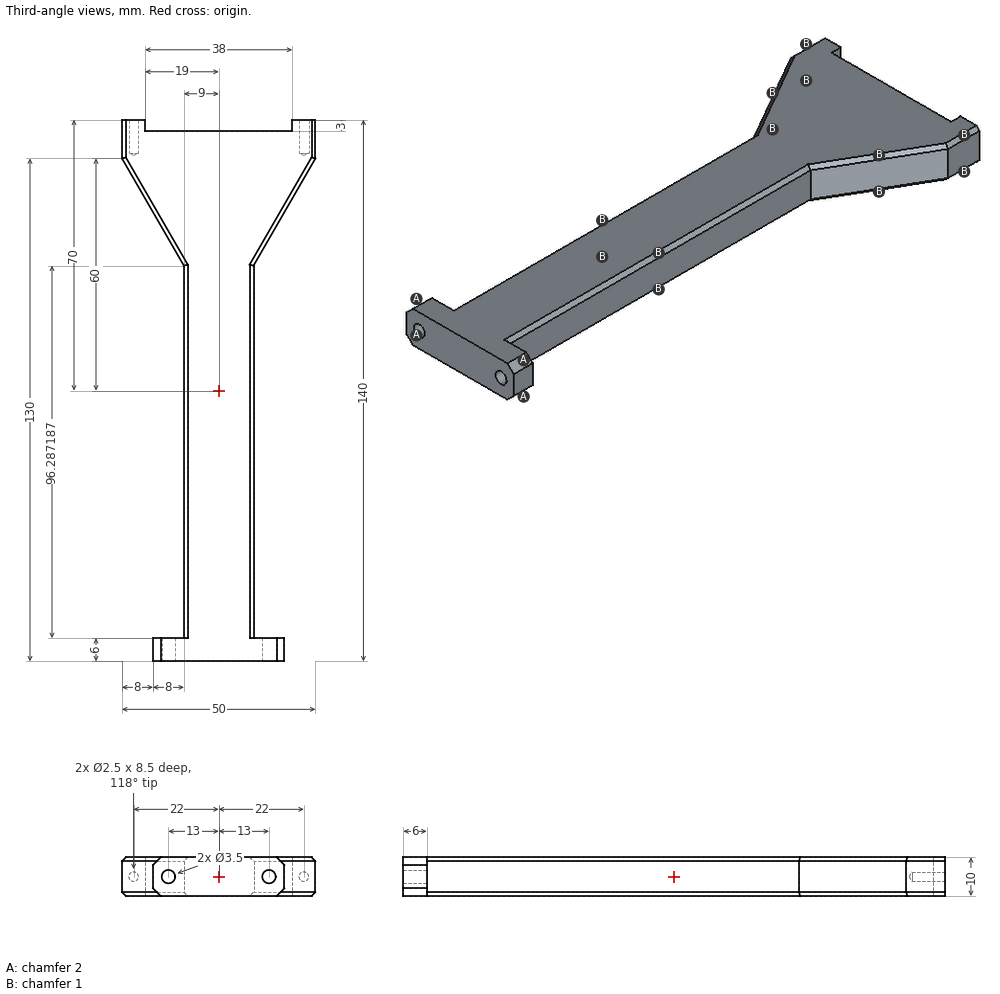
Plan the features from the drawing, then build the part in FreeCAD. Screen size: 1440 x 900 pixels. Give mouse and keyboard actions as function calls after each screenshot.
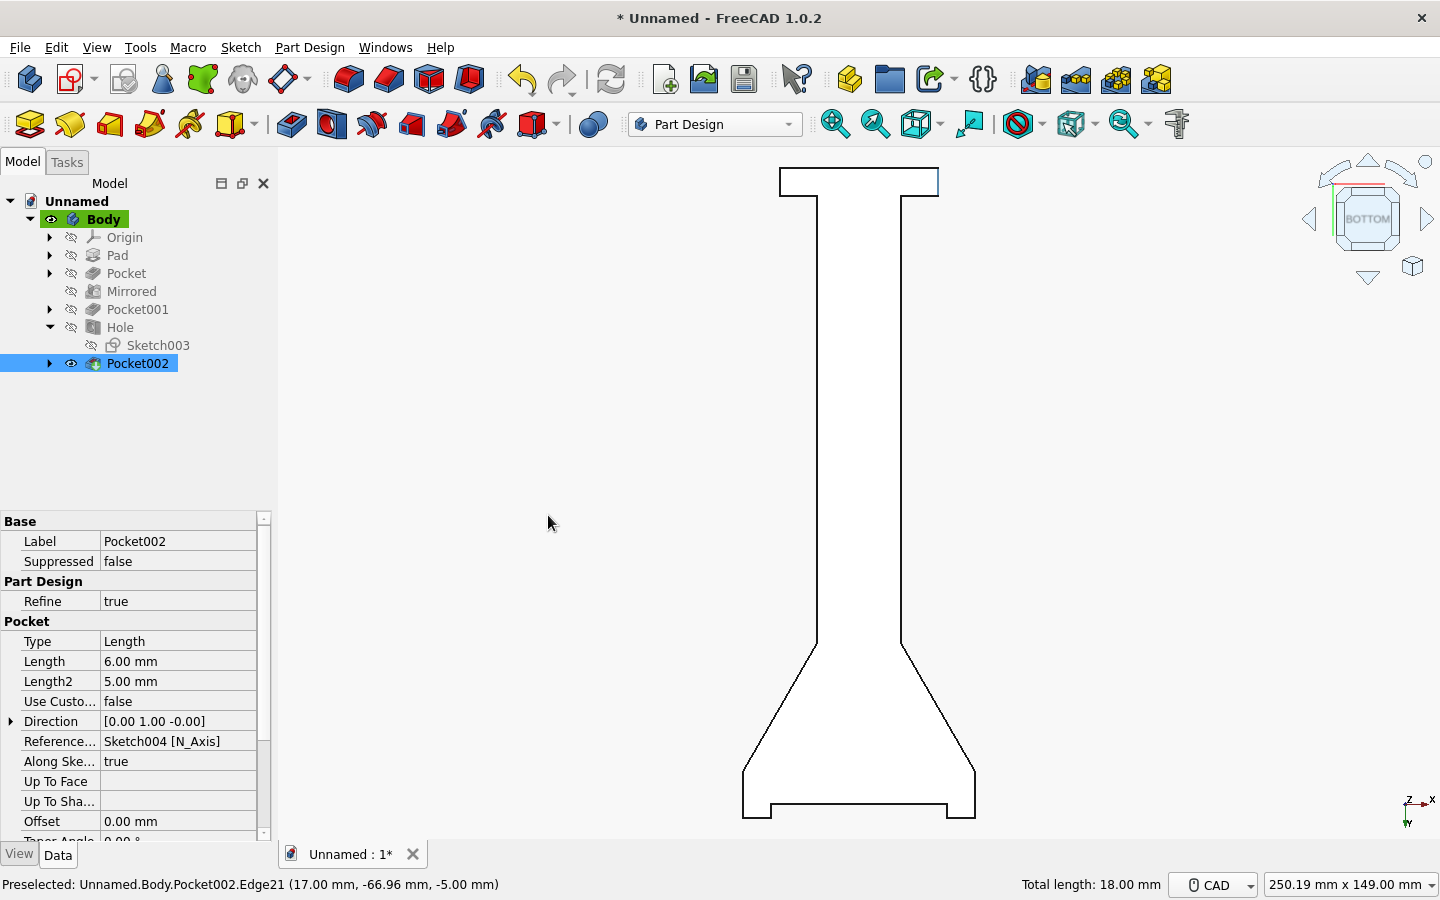
click(780, 181, ctrl)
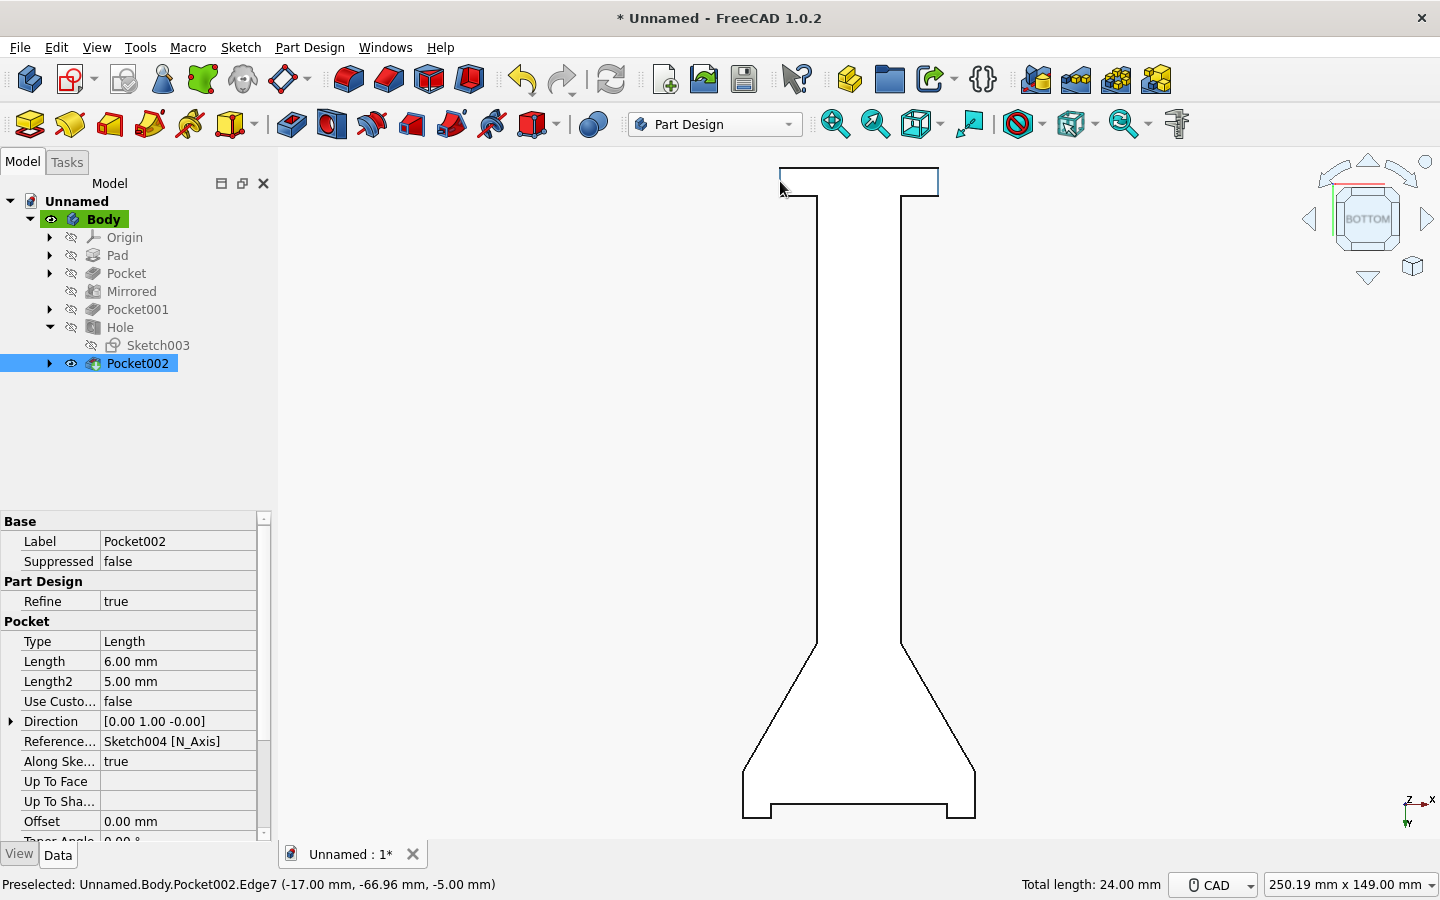
click(390, 80)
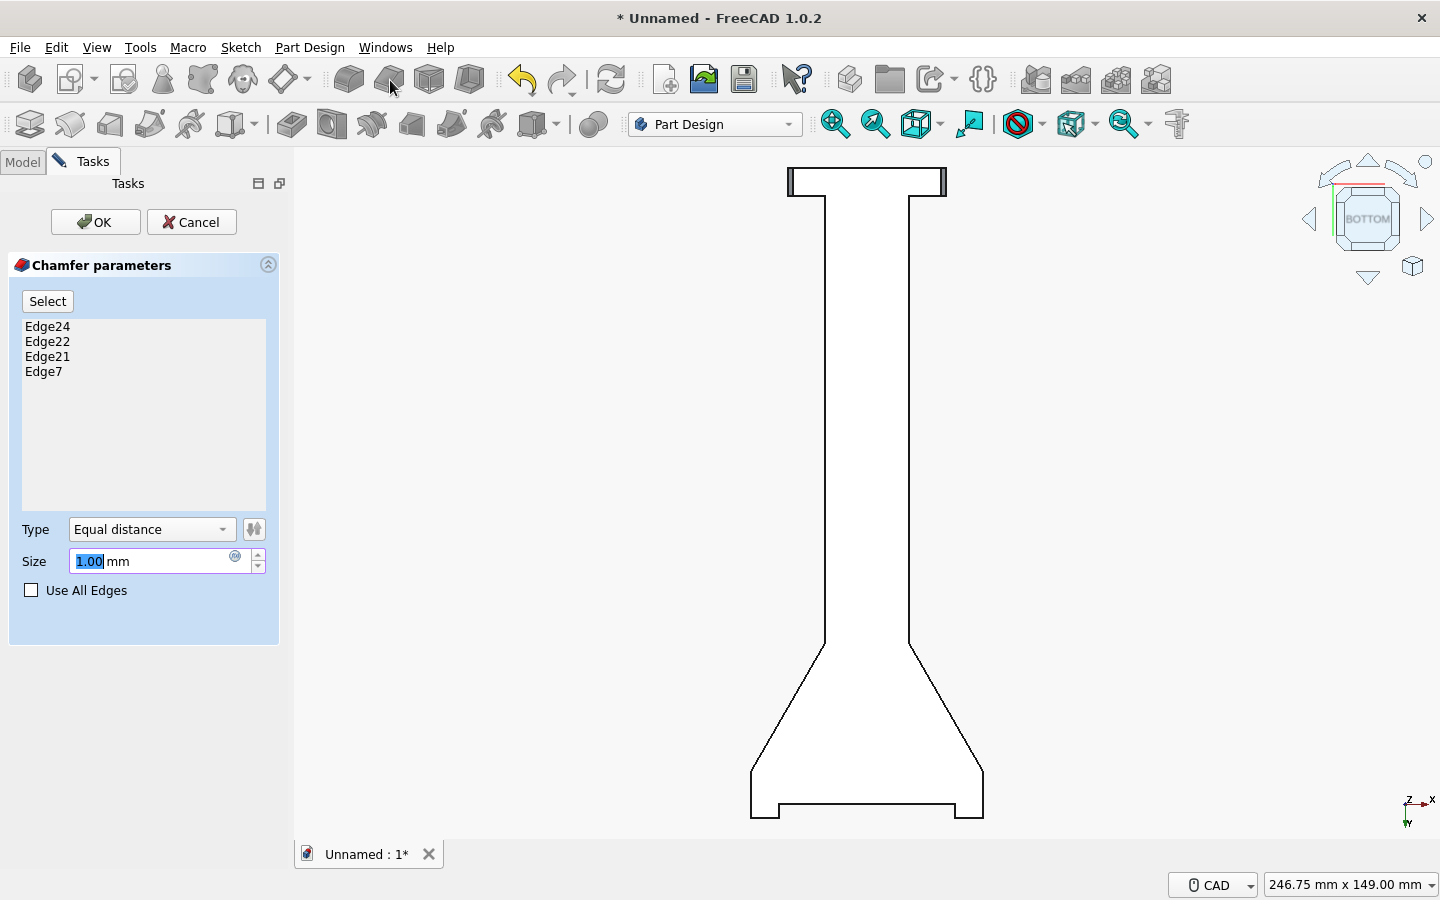
text(2)
key(Tab)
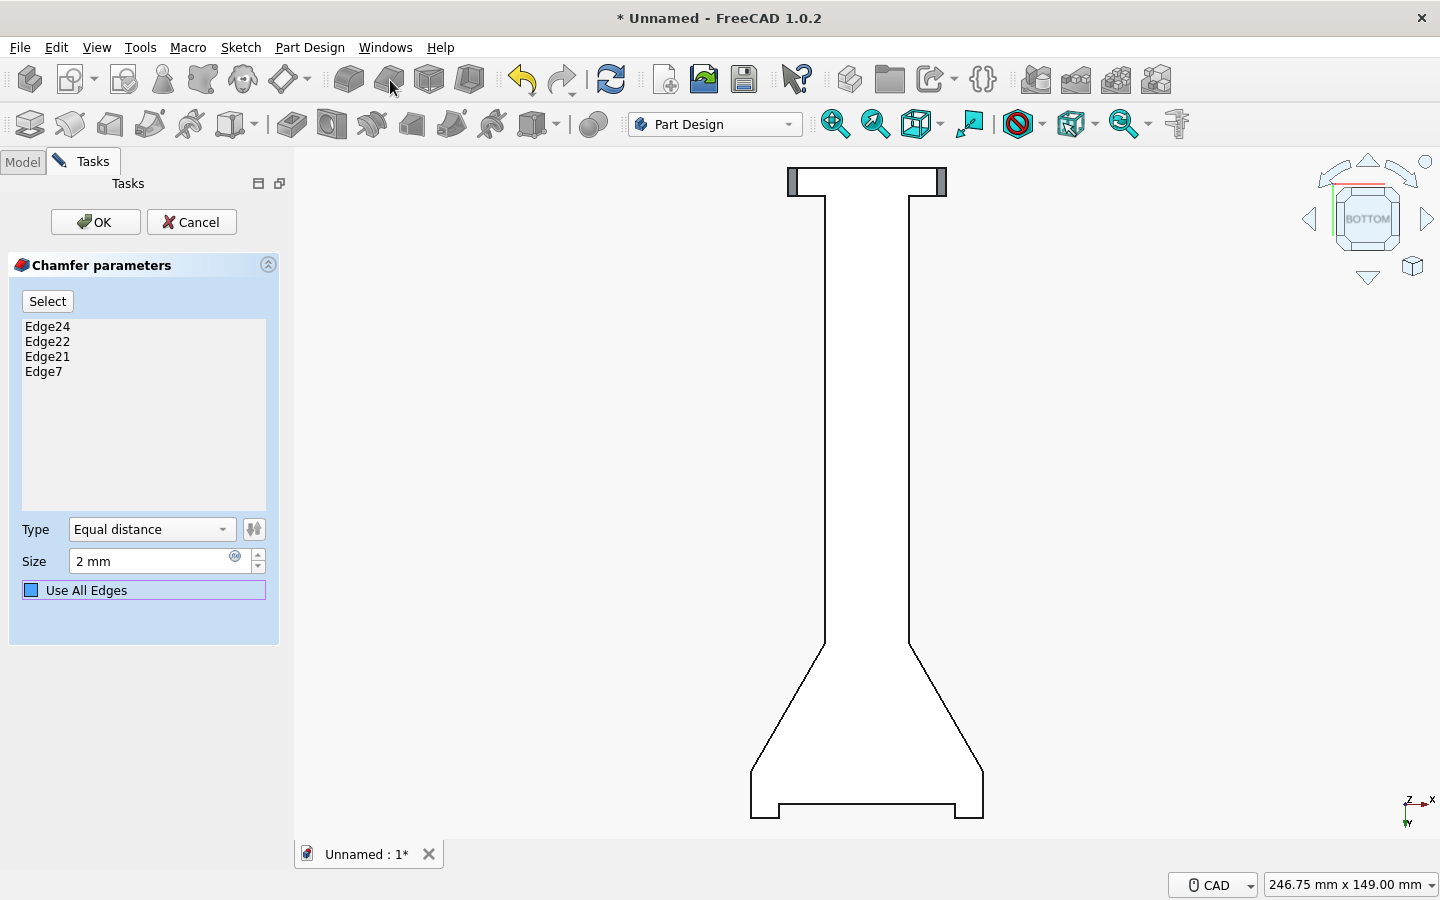
click(96, 222)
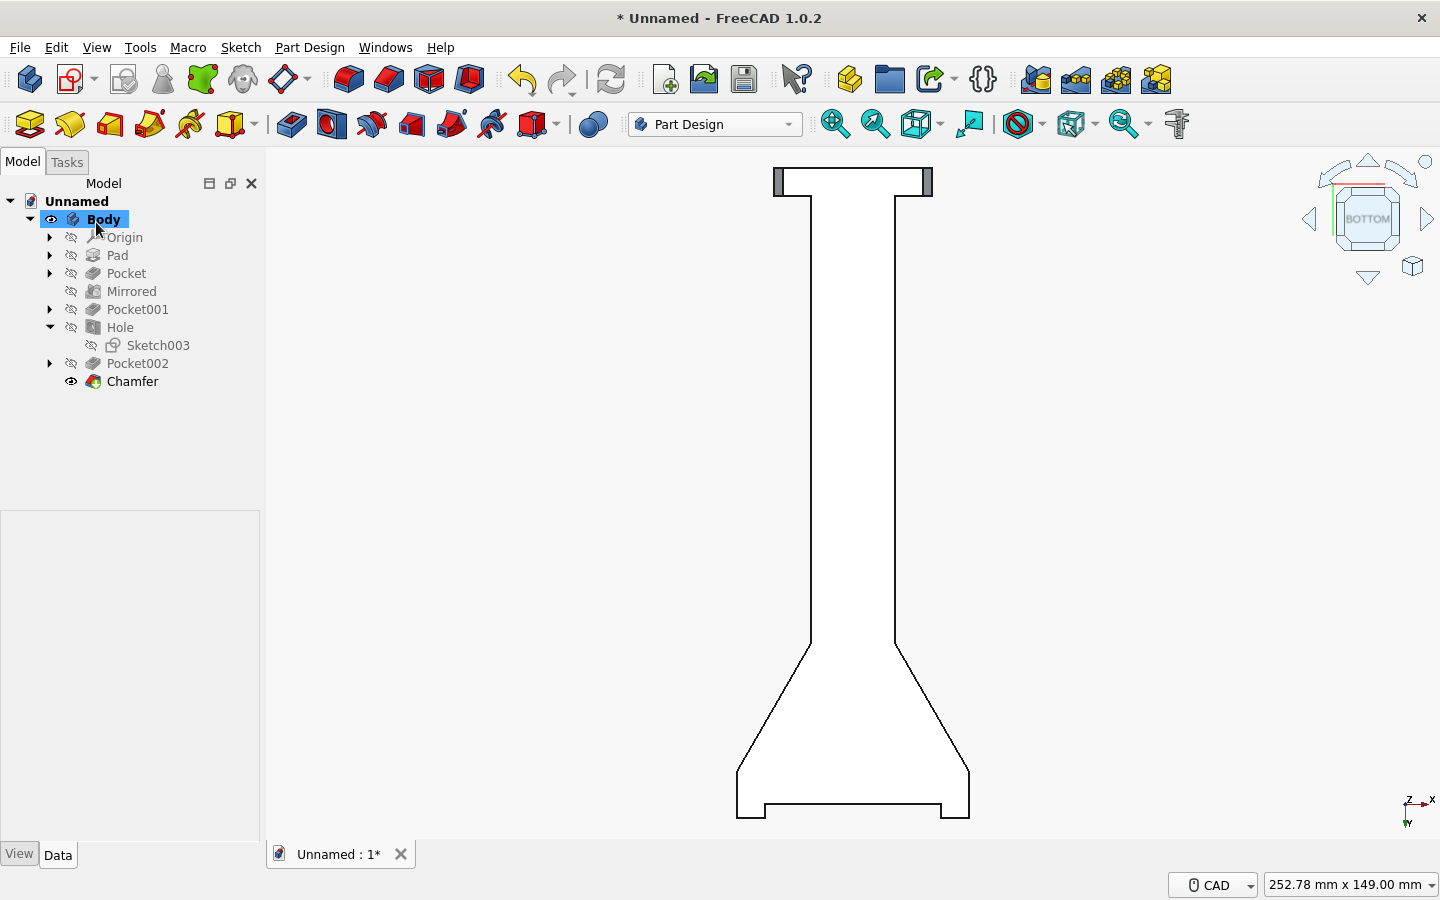
click(774, 706)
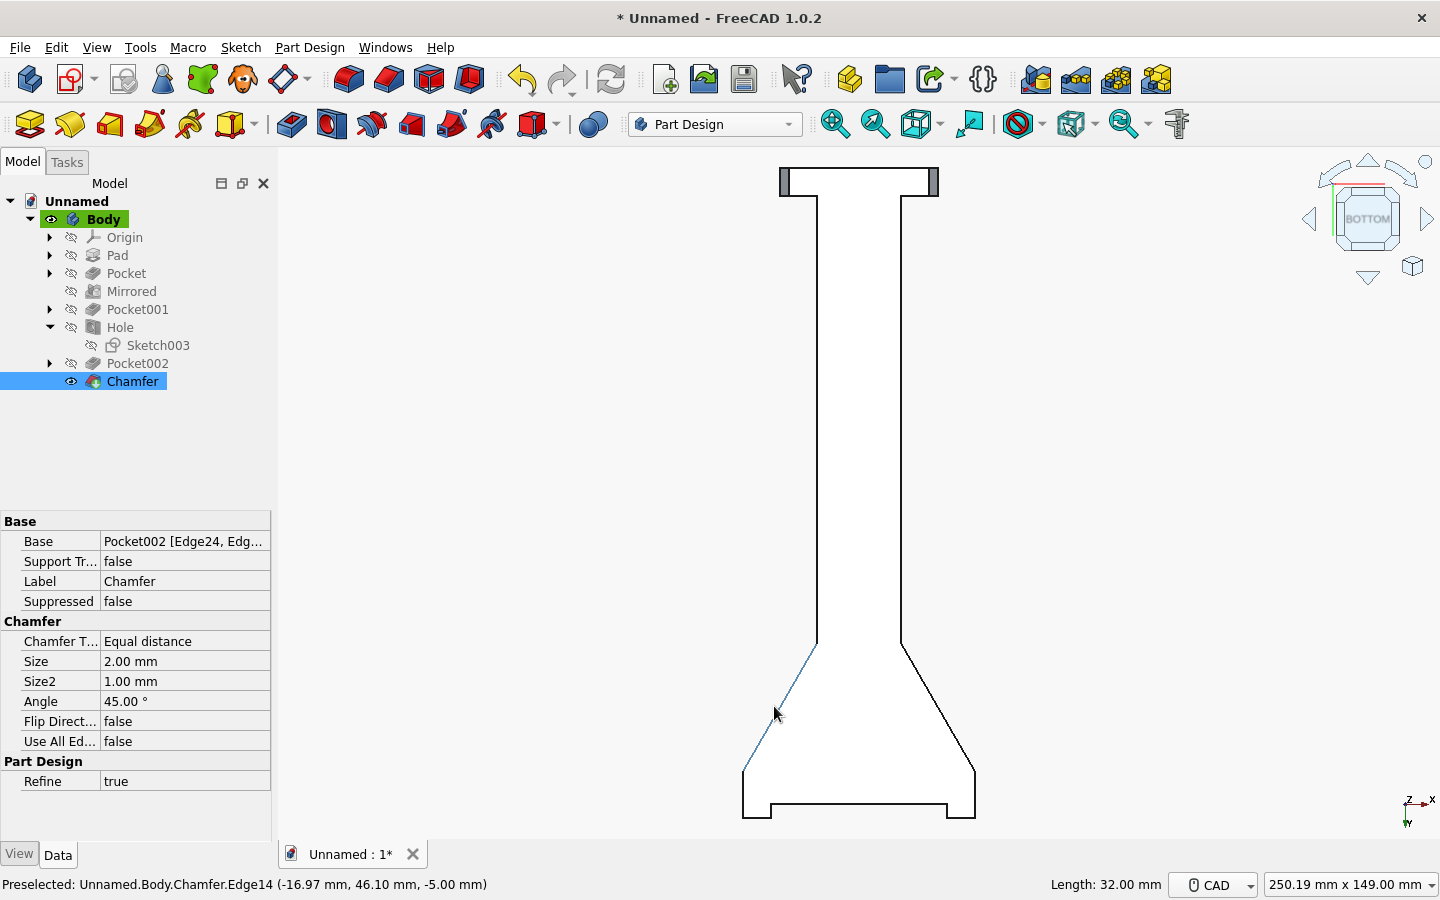
click(817, 418, ctrl)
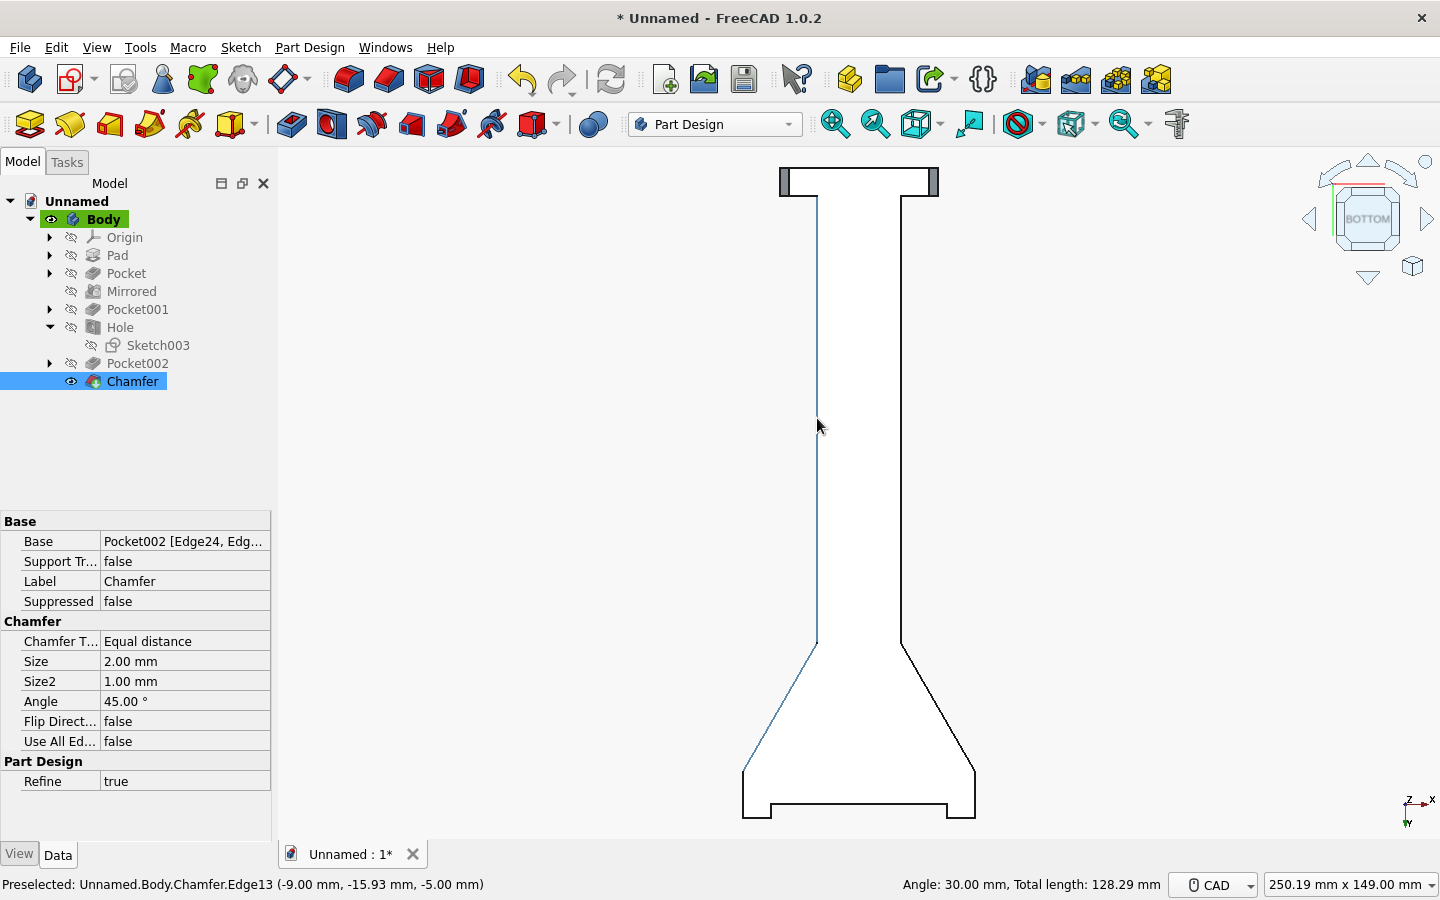
click(975, 794, ctrl)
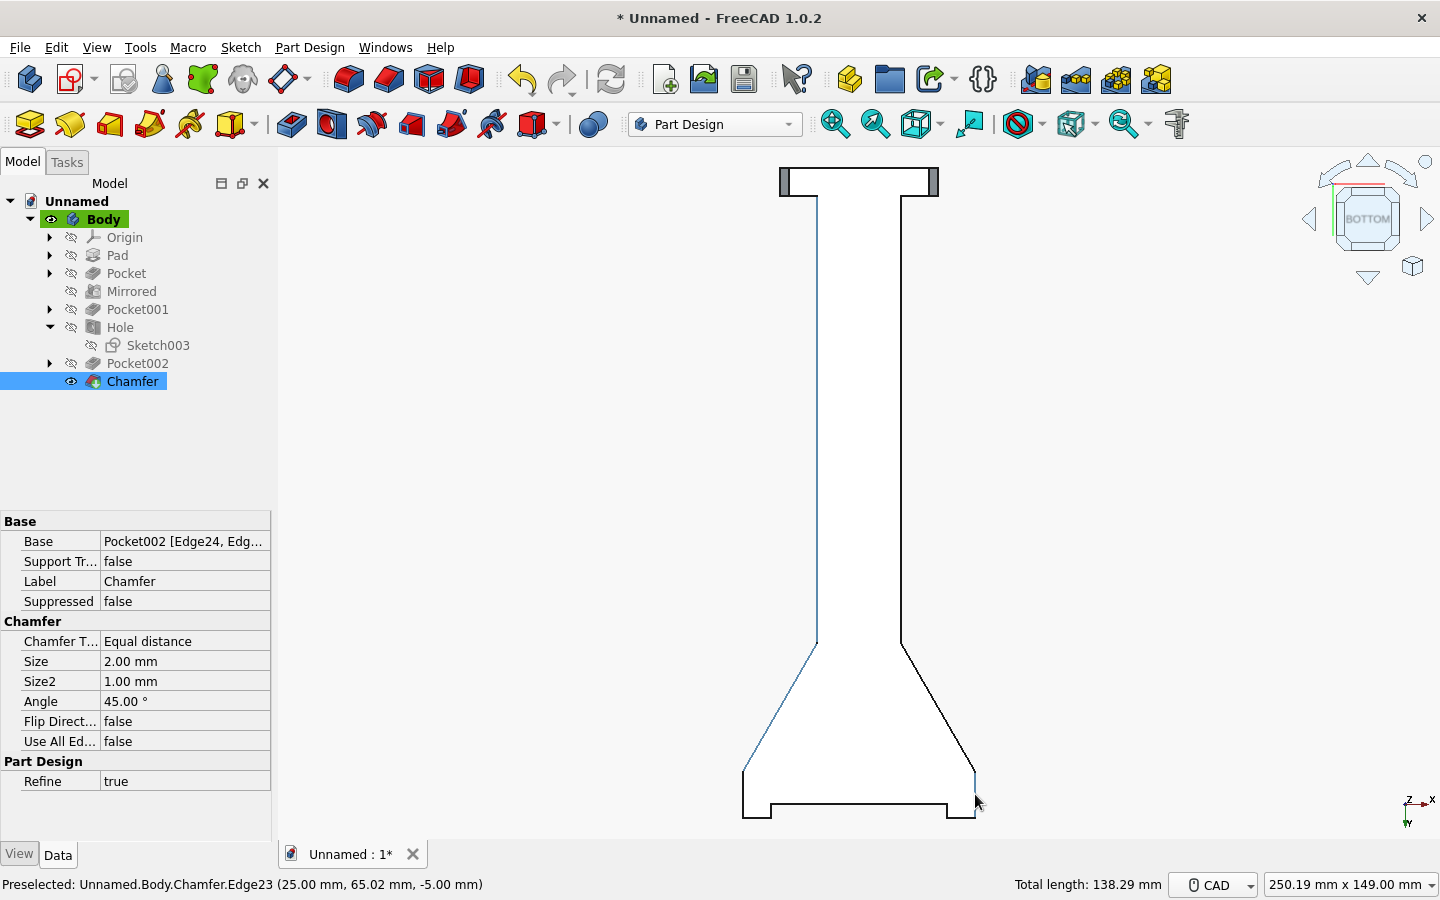
click(901, 418, ctrl)